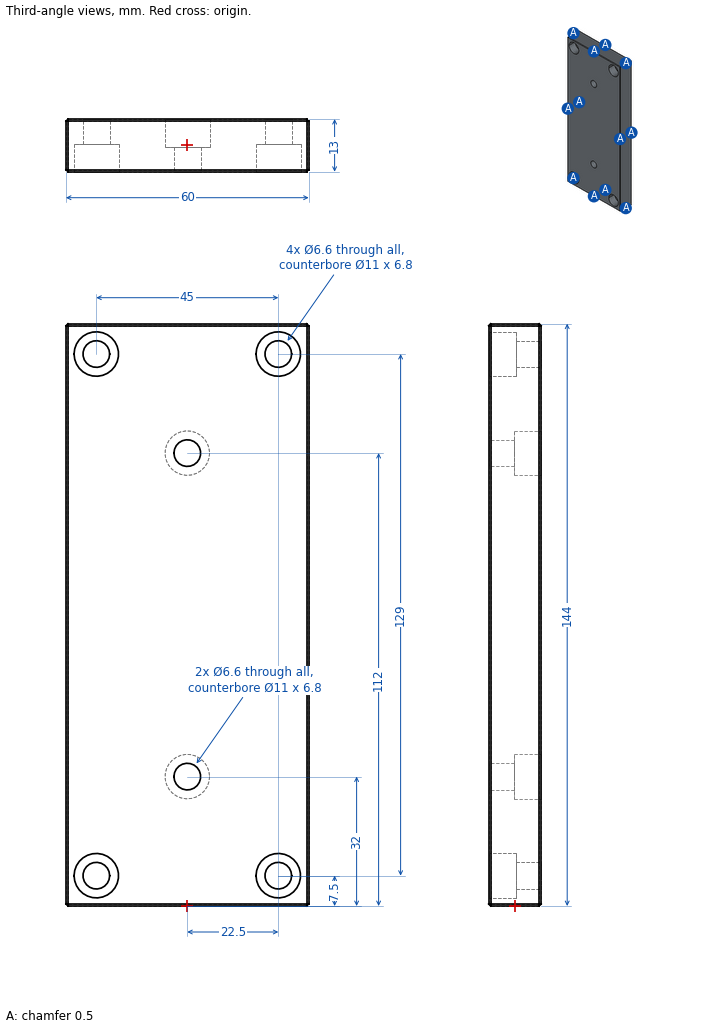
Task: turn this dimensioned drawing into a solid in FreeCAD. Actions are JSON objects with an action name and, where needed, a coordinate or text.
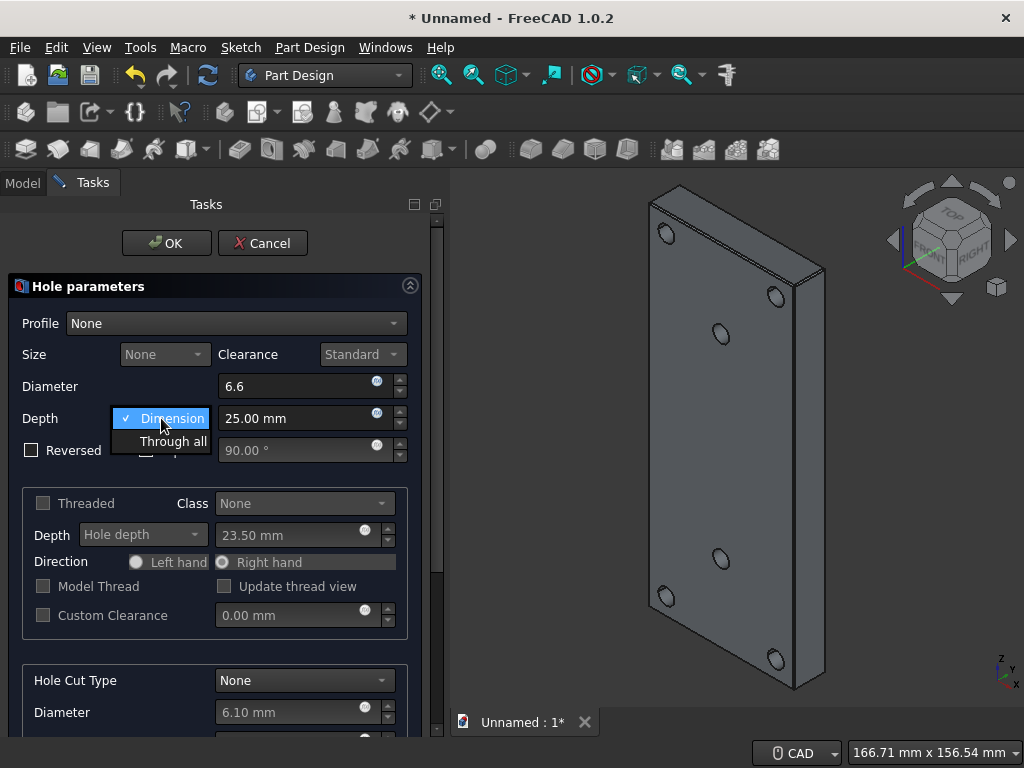
{"action": "left_click", "coordinate": [160, 442]}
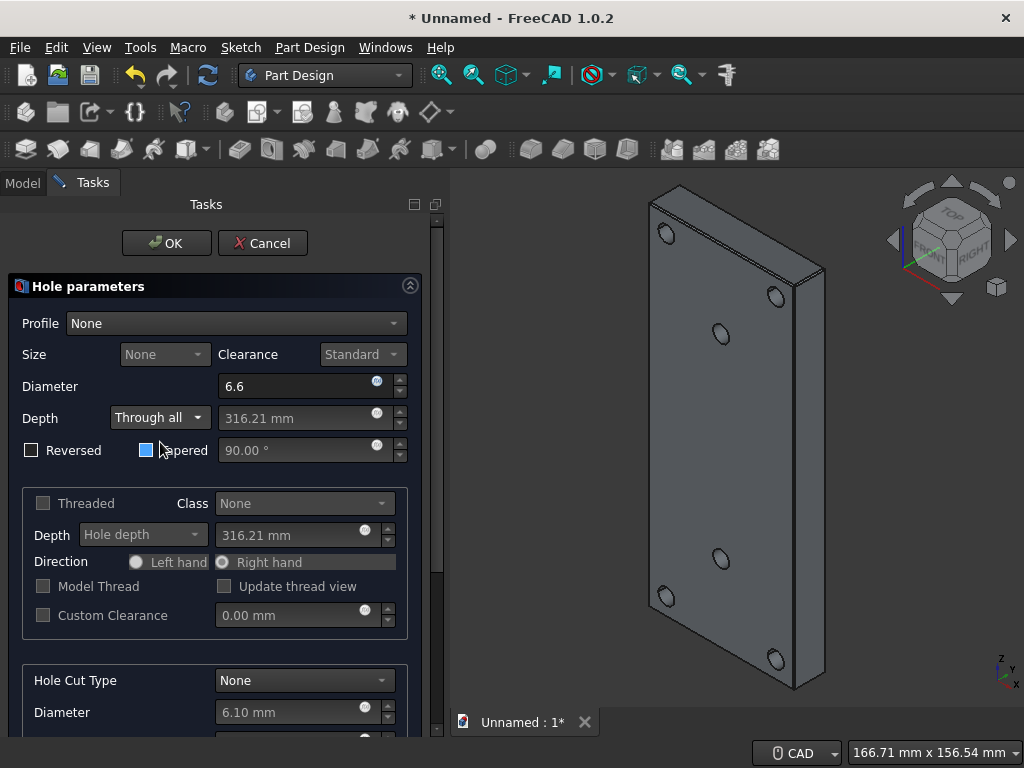
{"action": "left_click", "coordinate": [306, 680]}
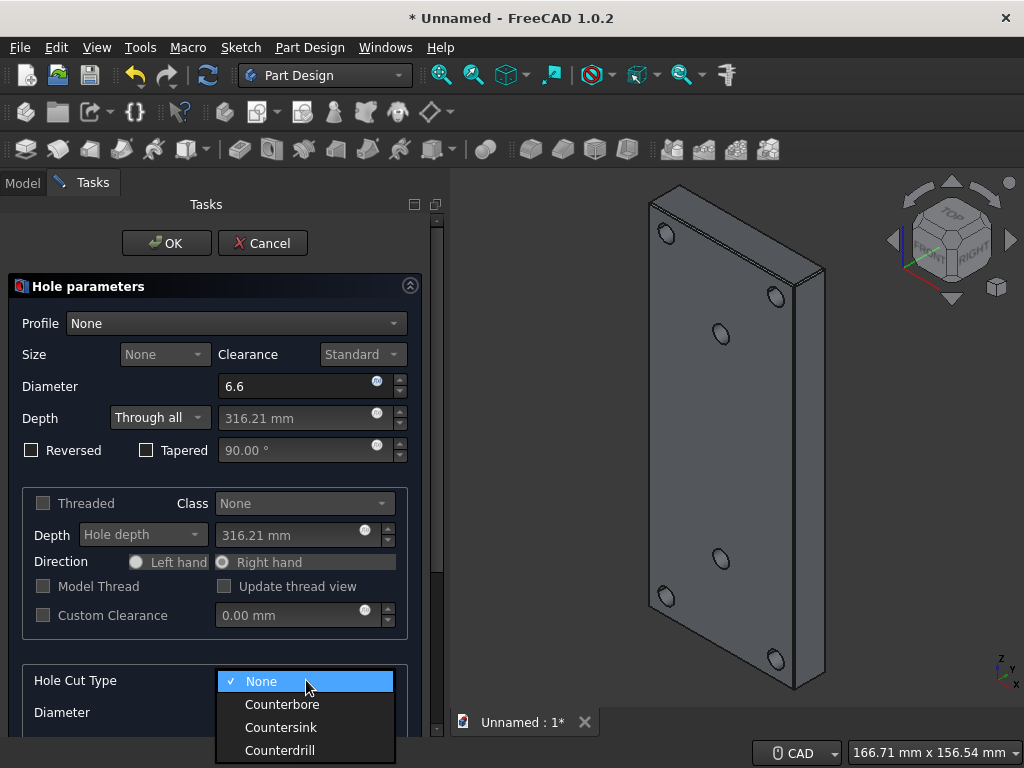
{"action": "left_click", "coordinate": [304, 704]}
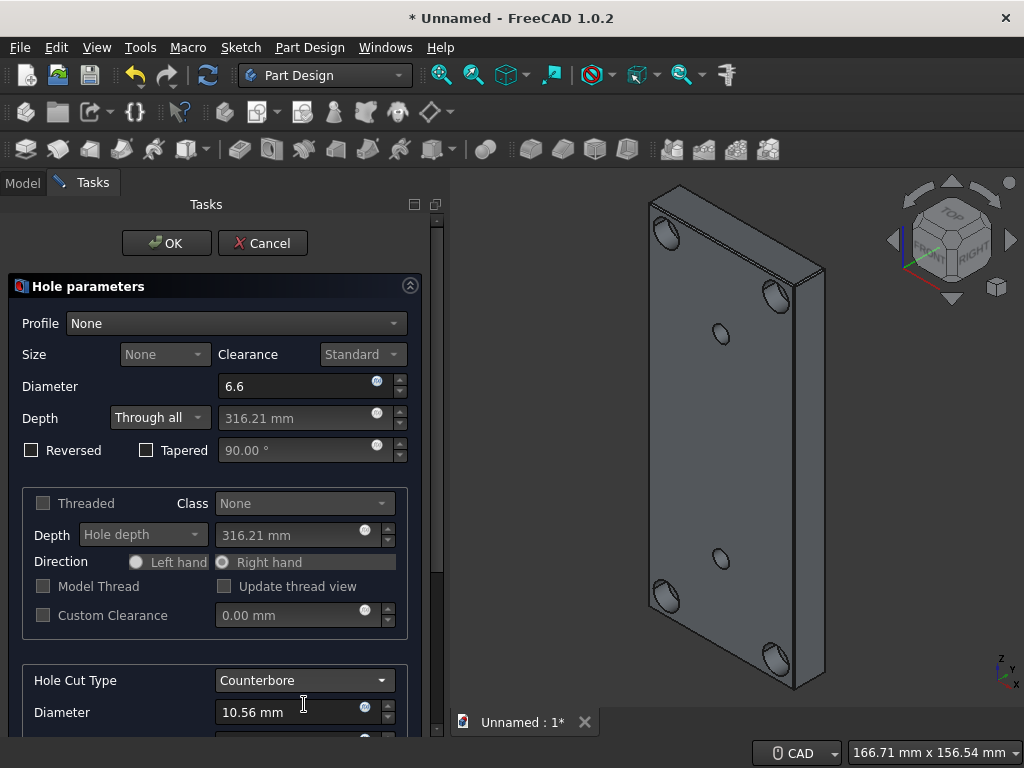
{"action": "triple_click", "coordinate": [298, 712]}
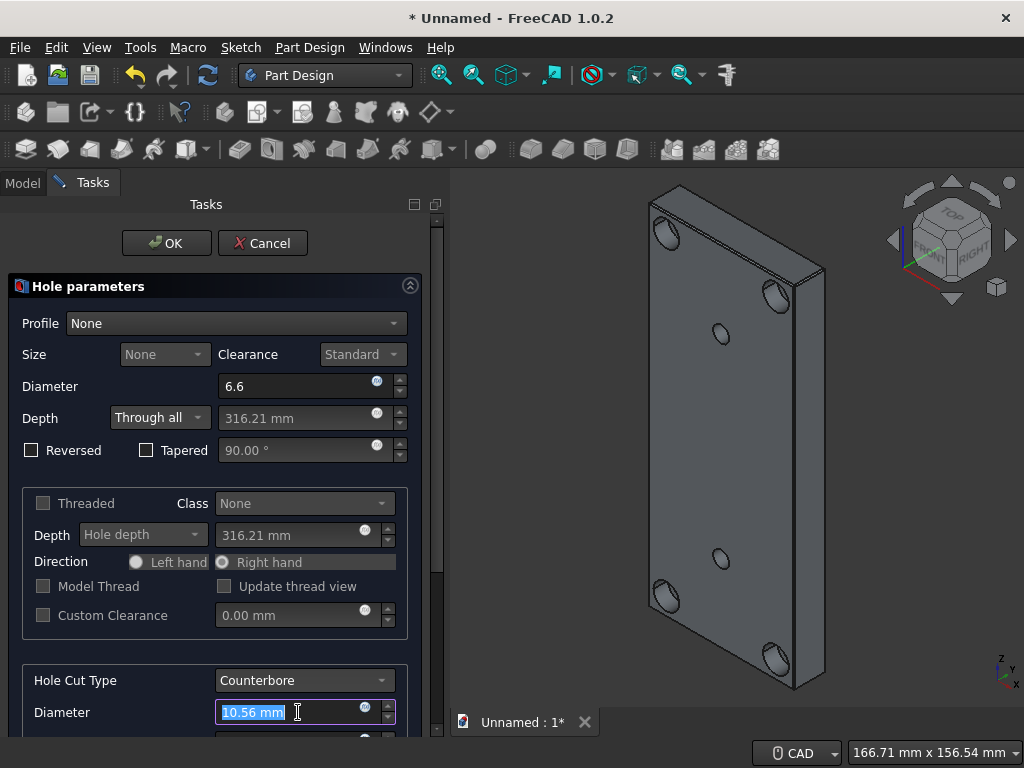
{"action": "type", "text": "11"}
{"action": "key", "text": "Tab"}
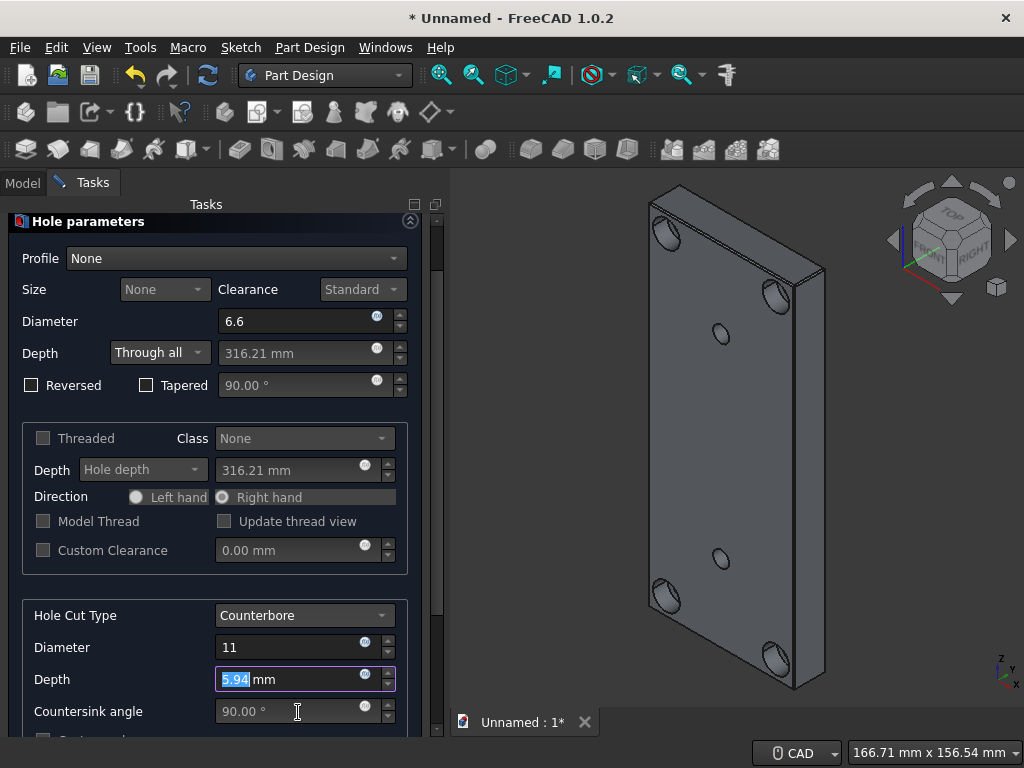
{"action": "type", "text": "6.8"}
{"action": "key", "text": "Tab"}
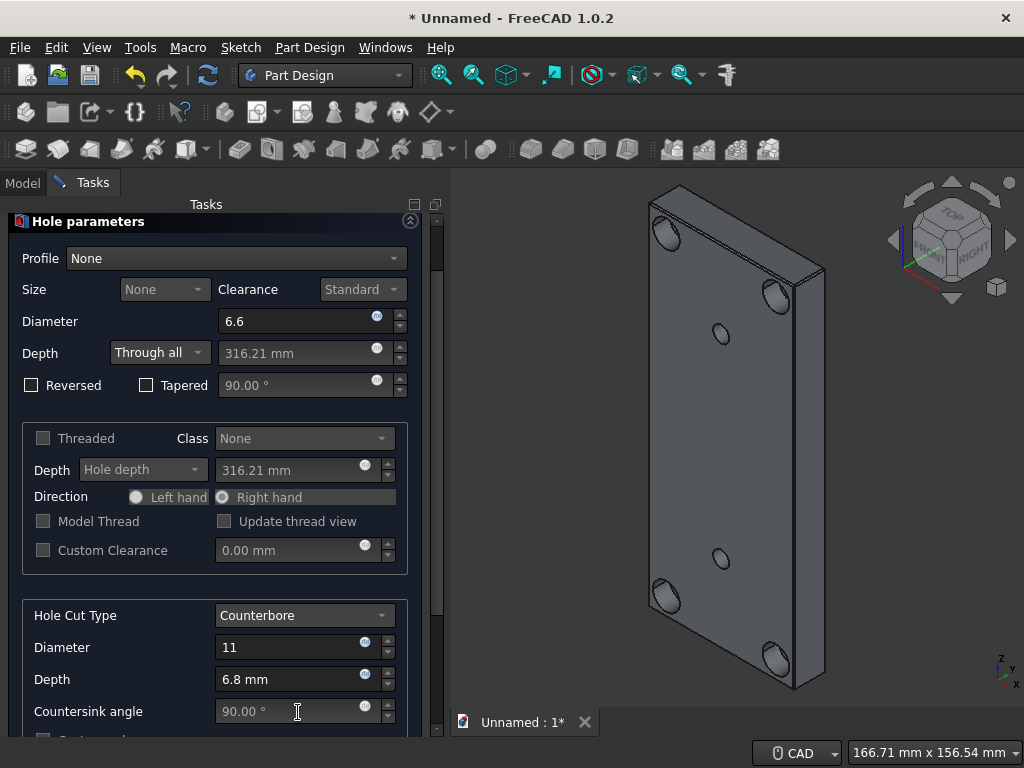
{"action": "scroll", "coordinate": [437, 475], "scroll_direction": "up", "scroll_amount": 2}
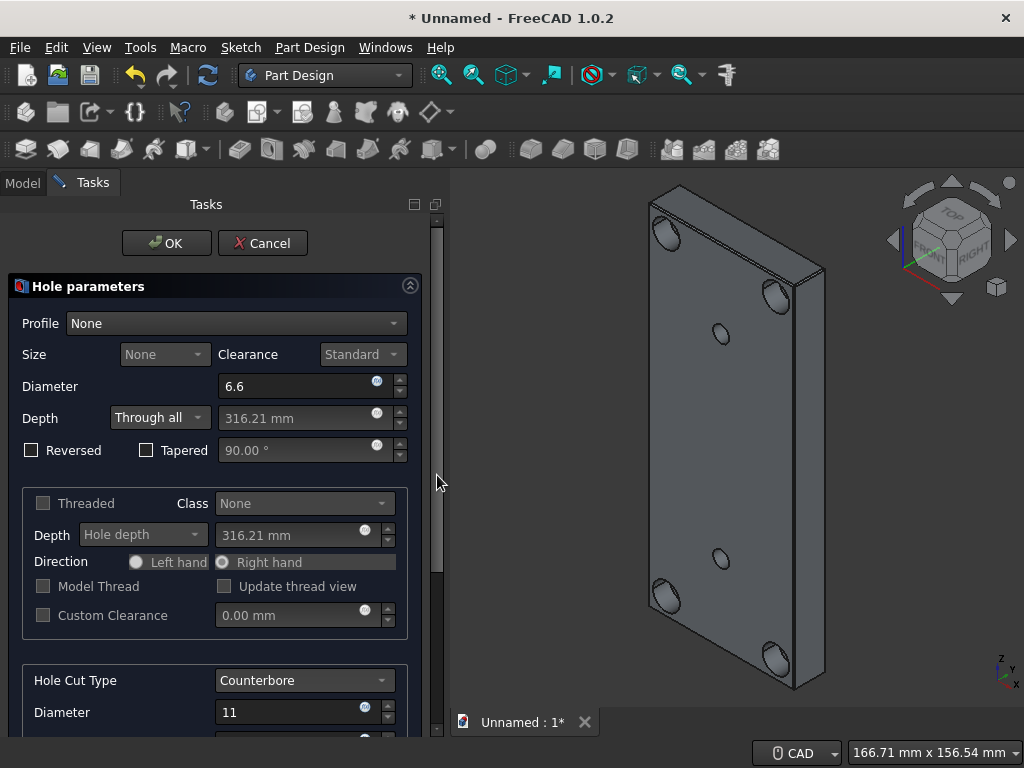
{"action": "left_click", "coordinate": [167, 243]}